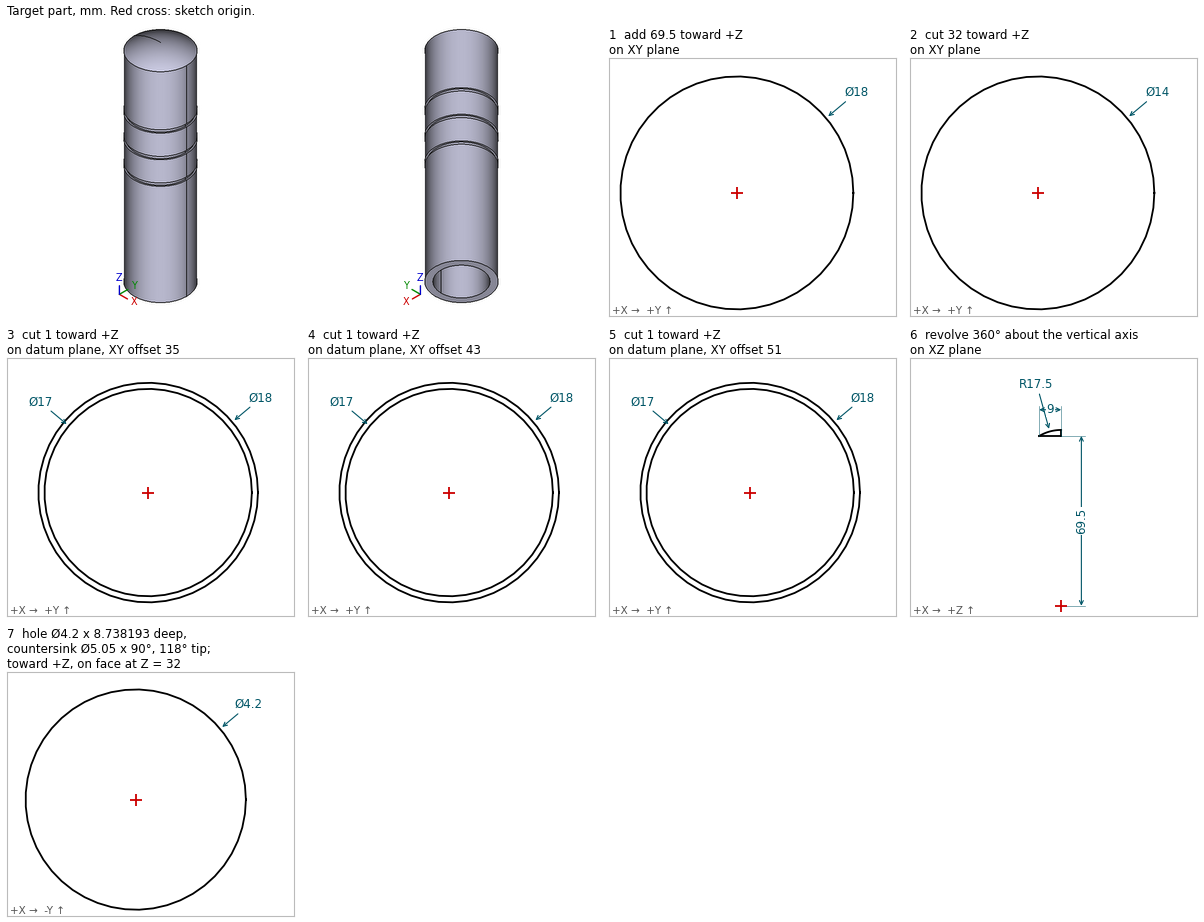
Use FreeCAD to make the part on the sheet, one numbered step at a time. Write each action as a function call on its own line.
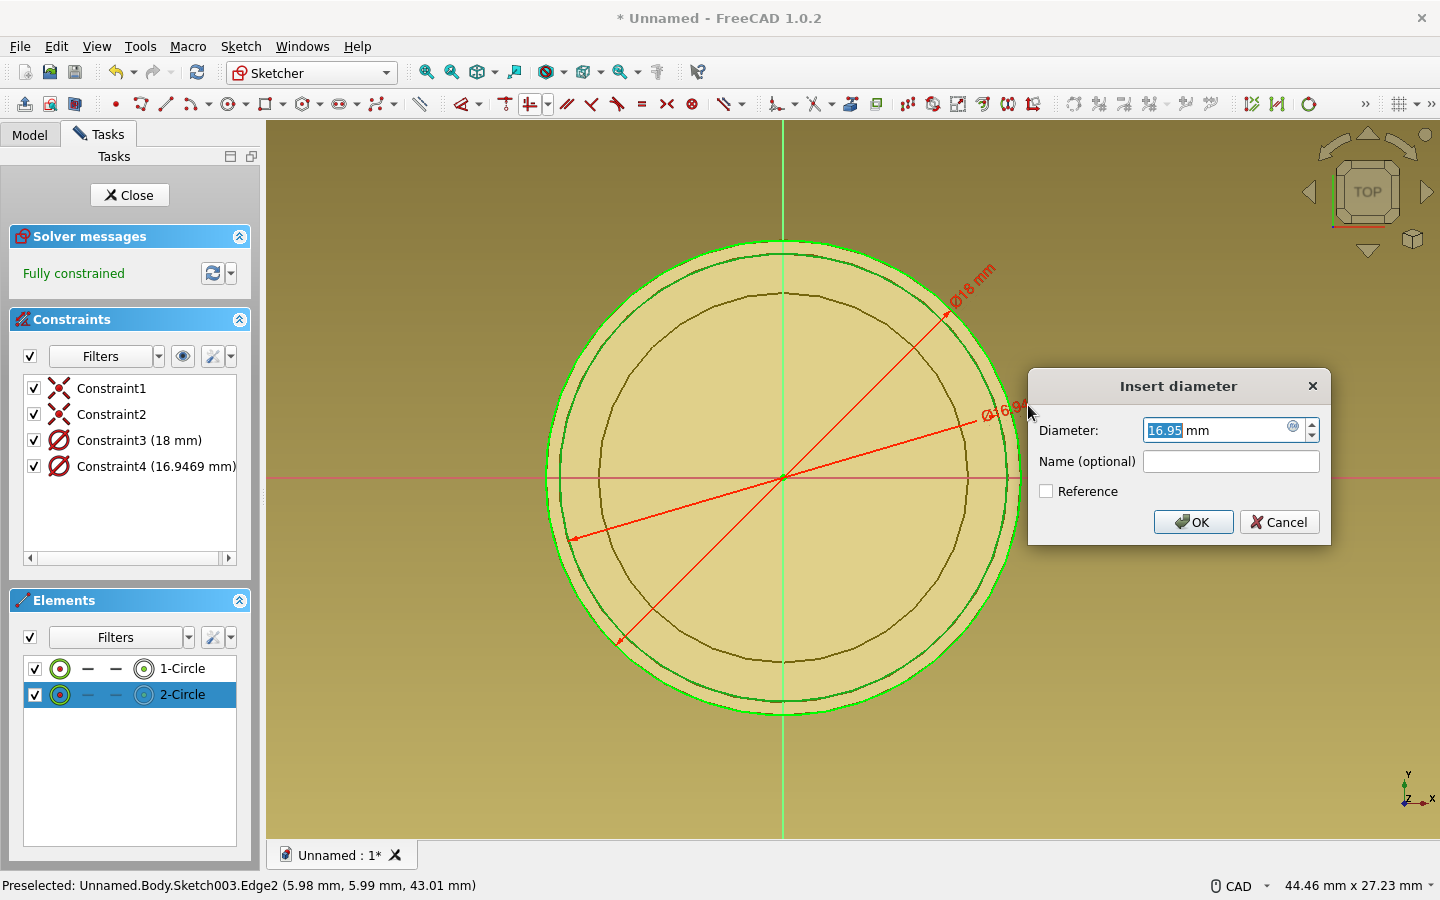
text(17)
key(Return)
key(Escape)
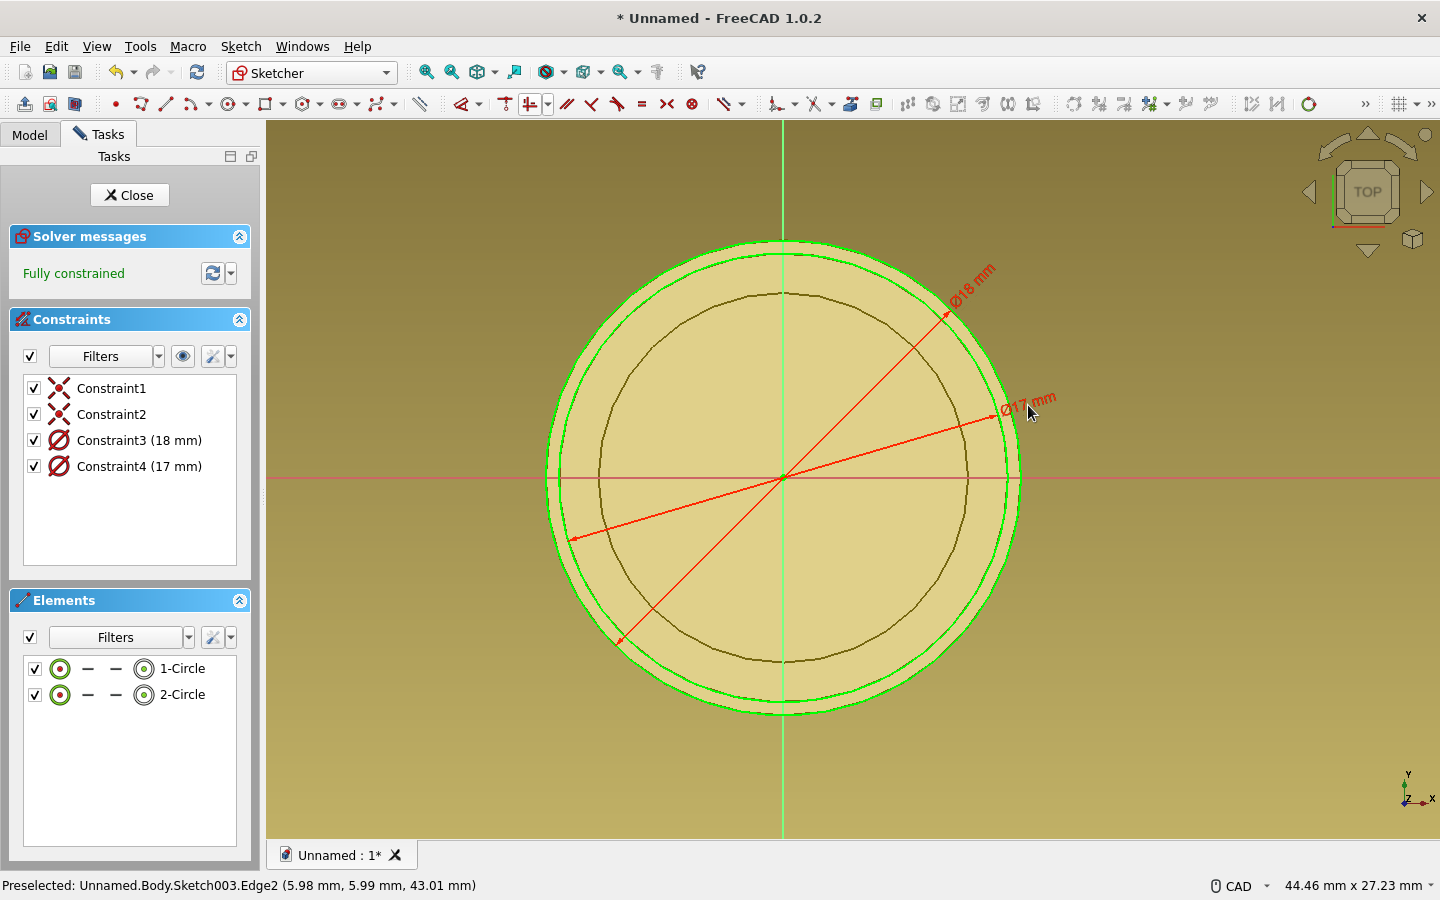
click(130, 195)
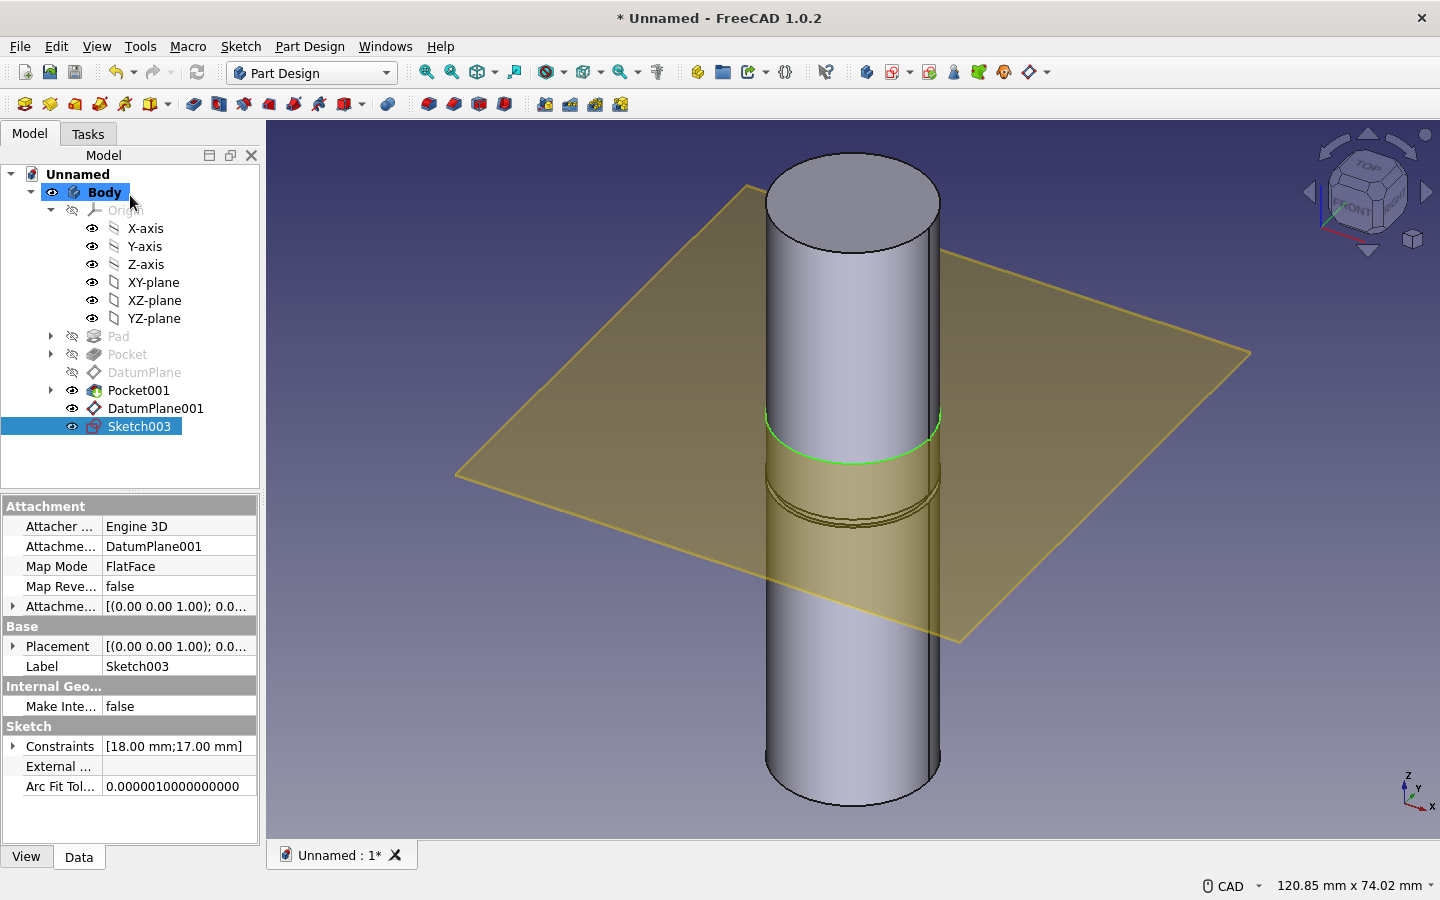
click(194, 104)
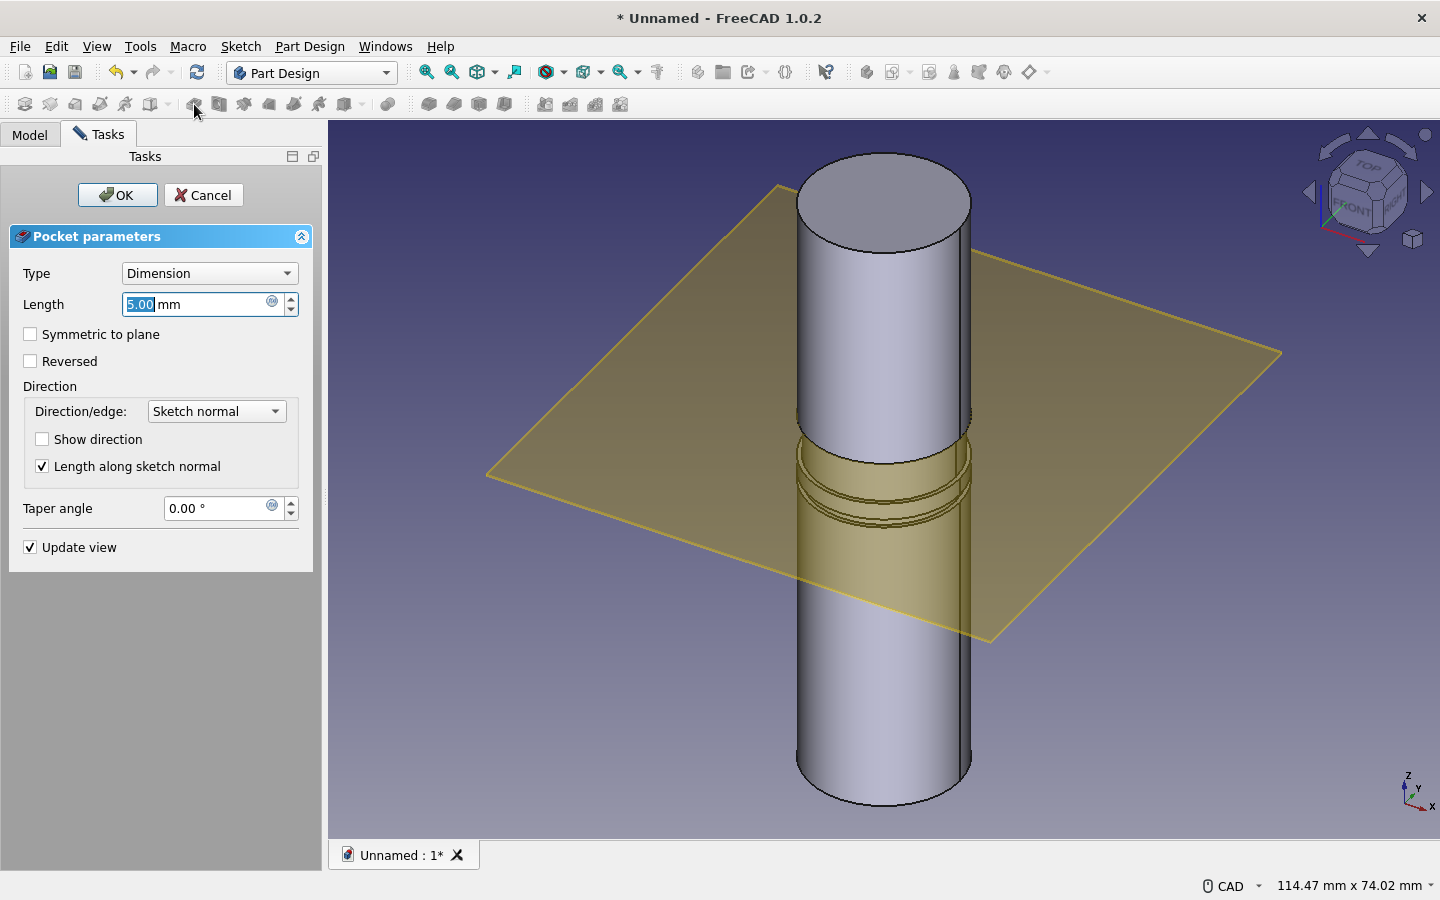
text(1)
key(Tab)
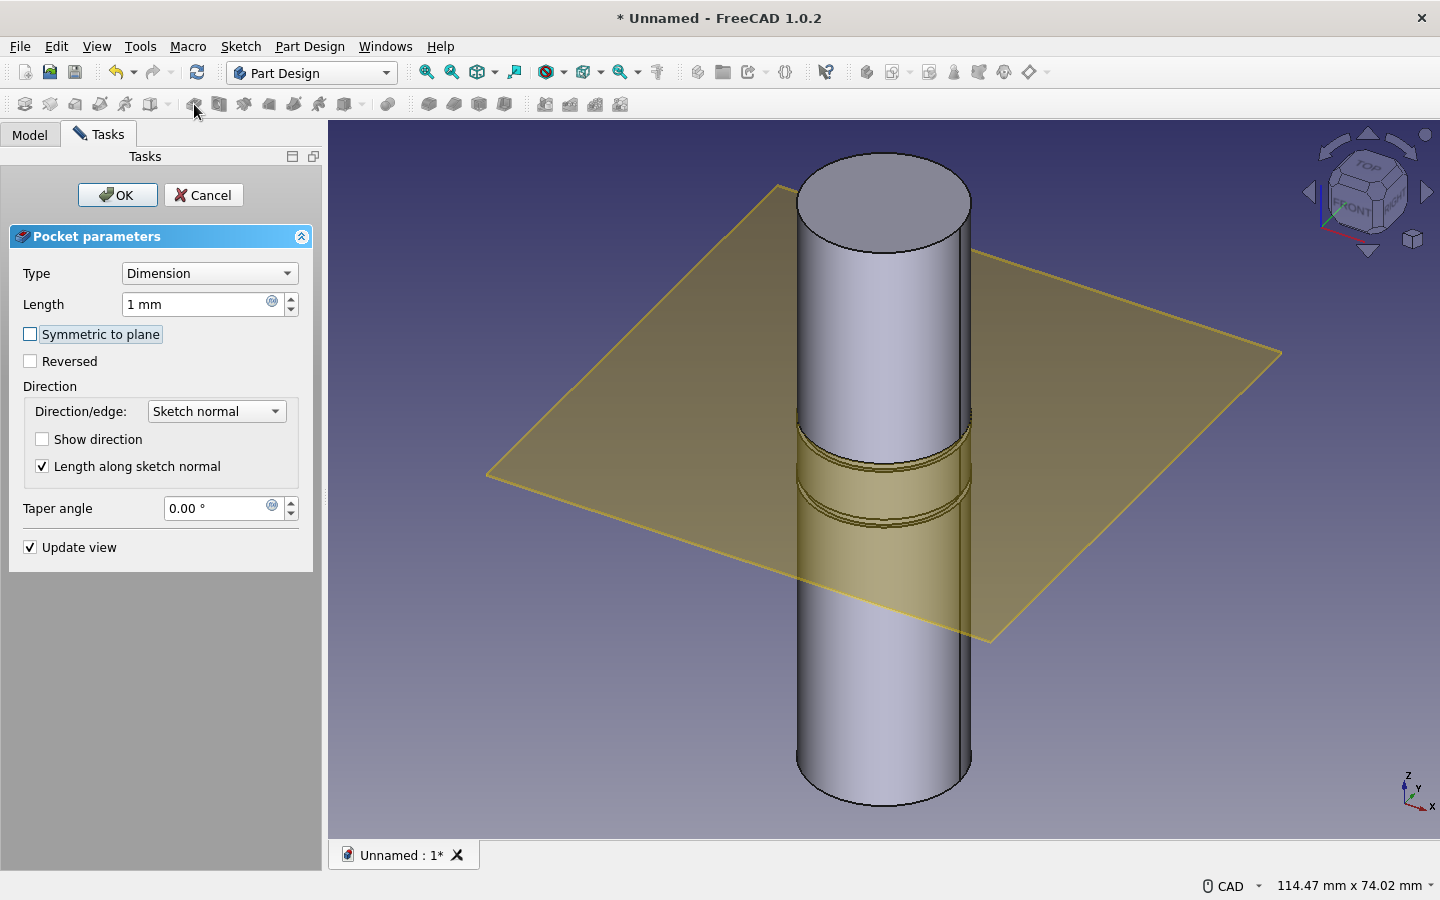
click(31, 361)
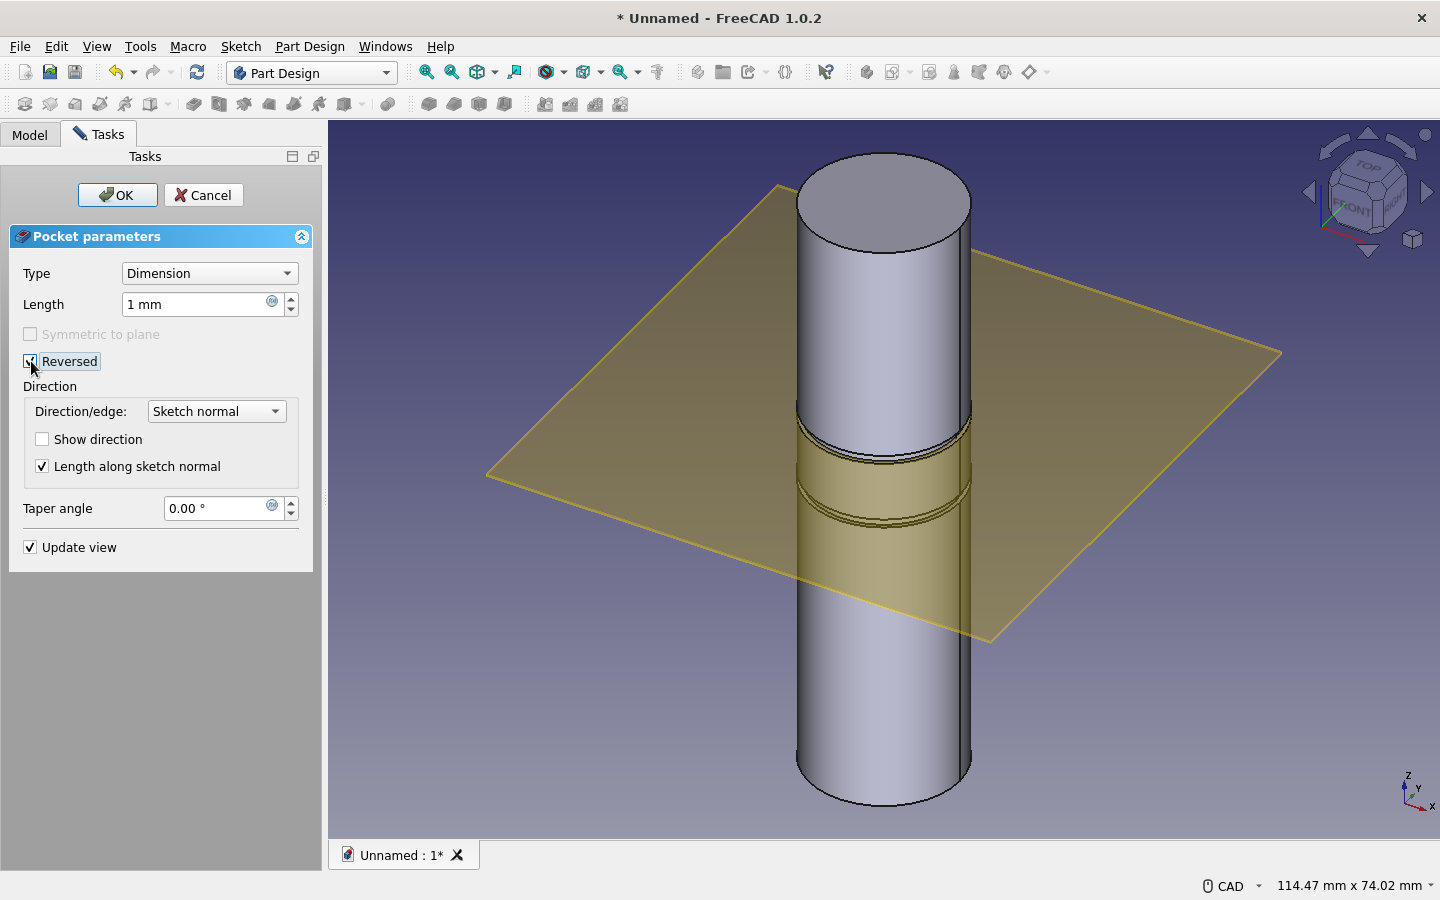
click(118, 195)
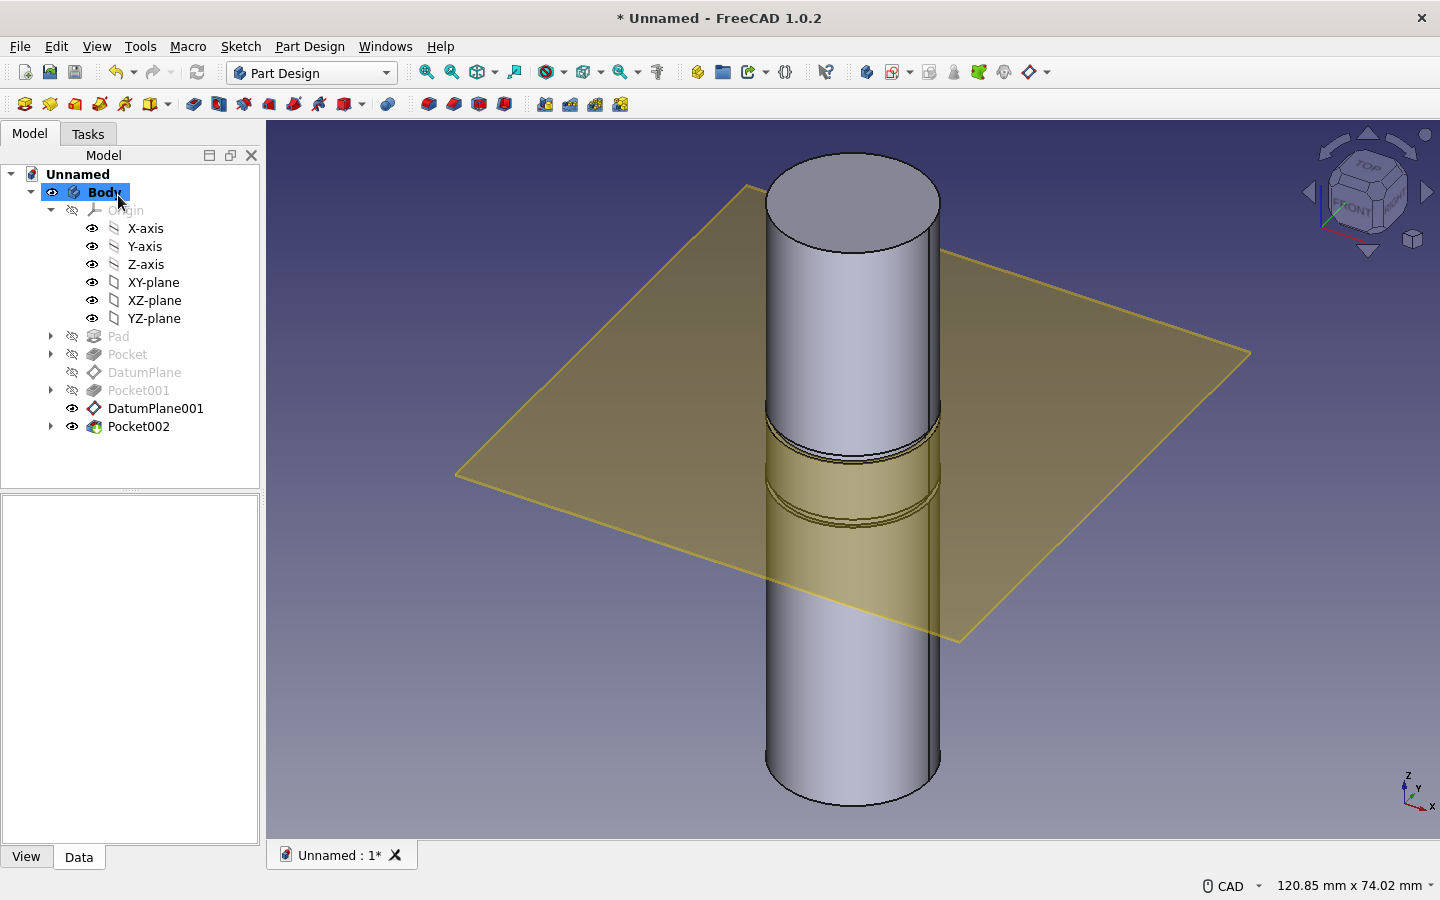
click(117, 408)
key(space)